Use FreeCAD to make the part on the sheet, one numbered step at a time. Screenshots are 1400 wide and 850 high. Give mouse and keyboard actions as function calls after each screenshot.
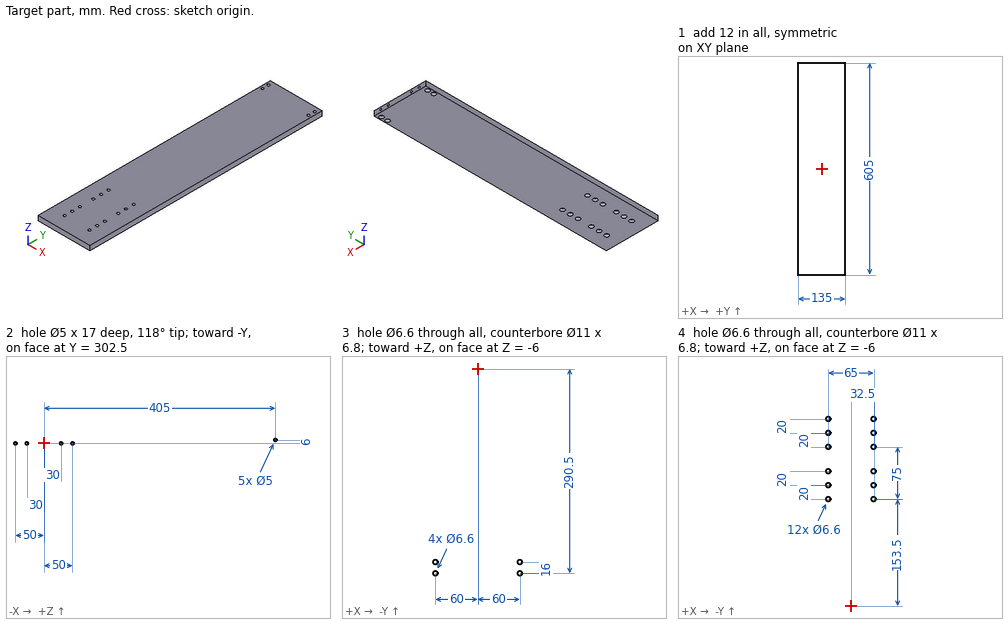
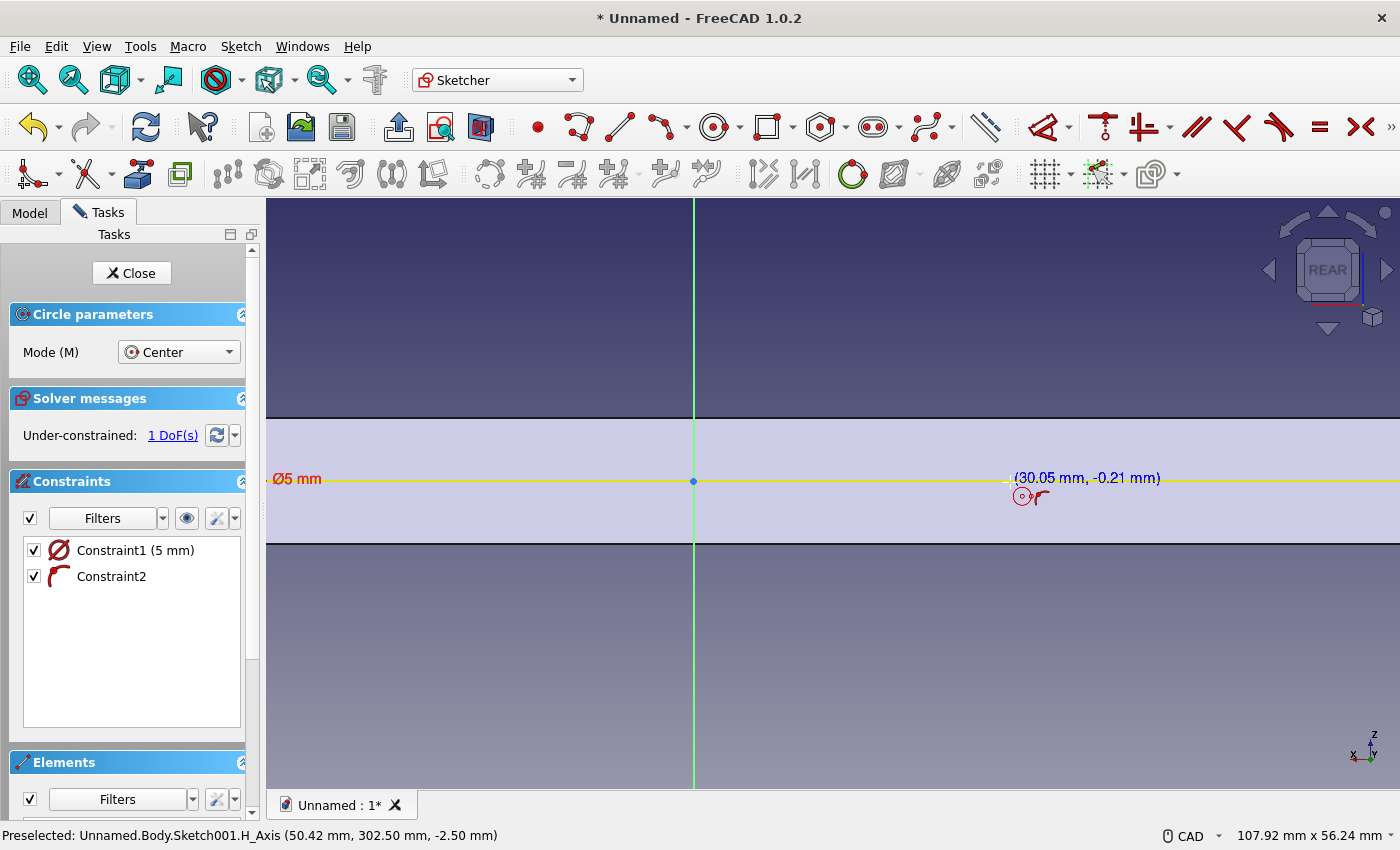
scroll(484, 500, down, 10)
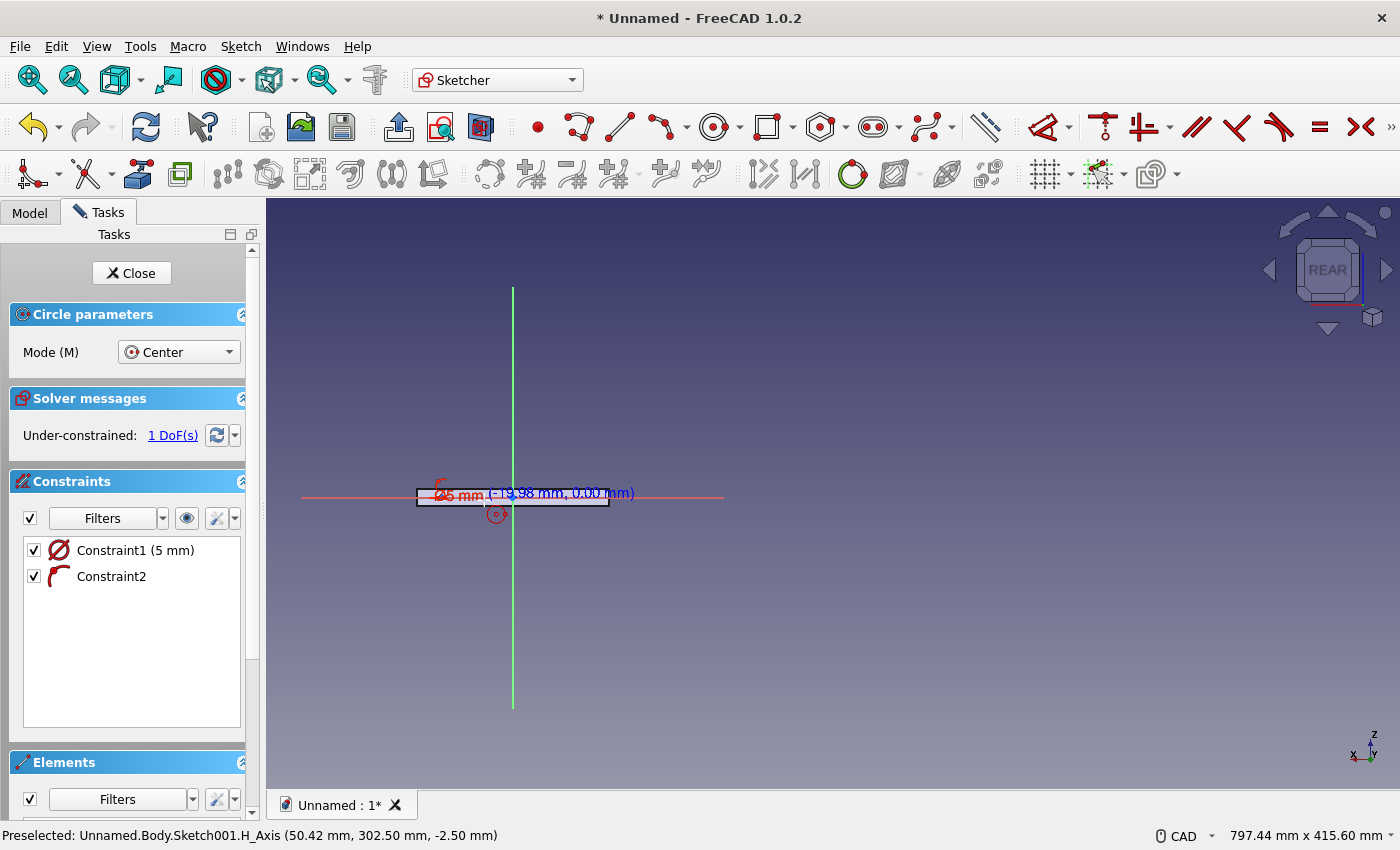
click(555, 498)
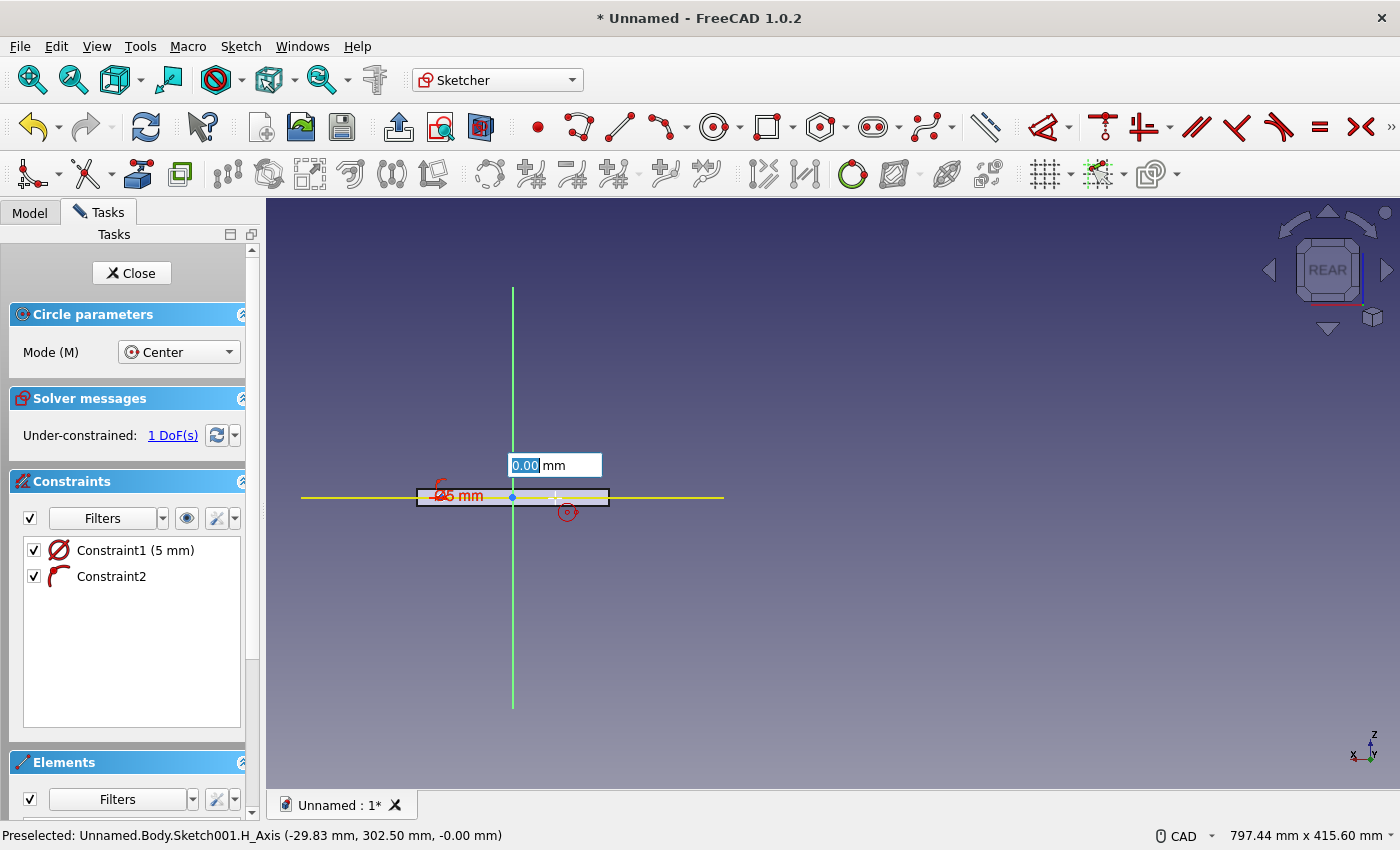
scroll(554, 501, up, 8)
move(553, 500)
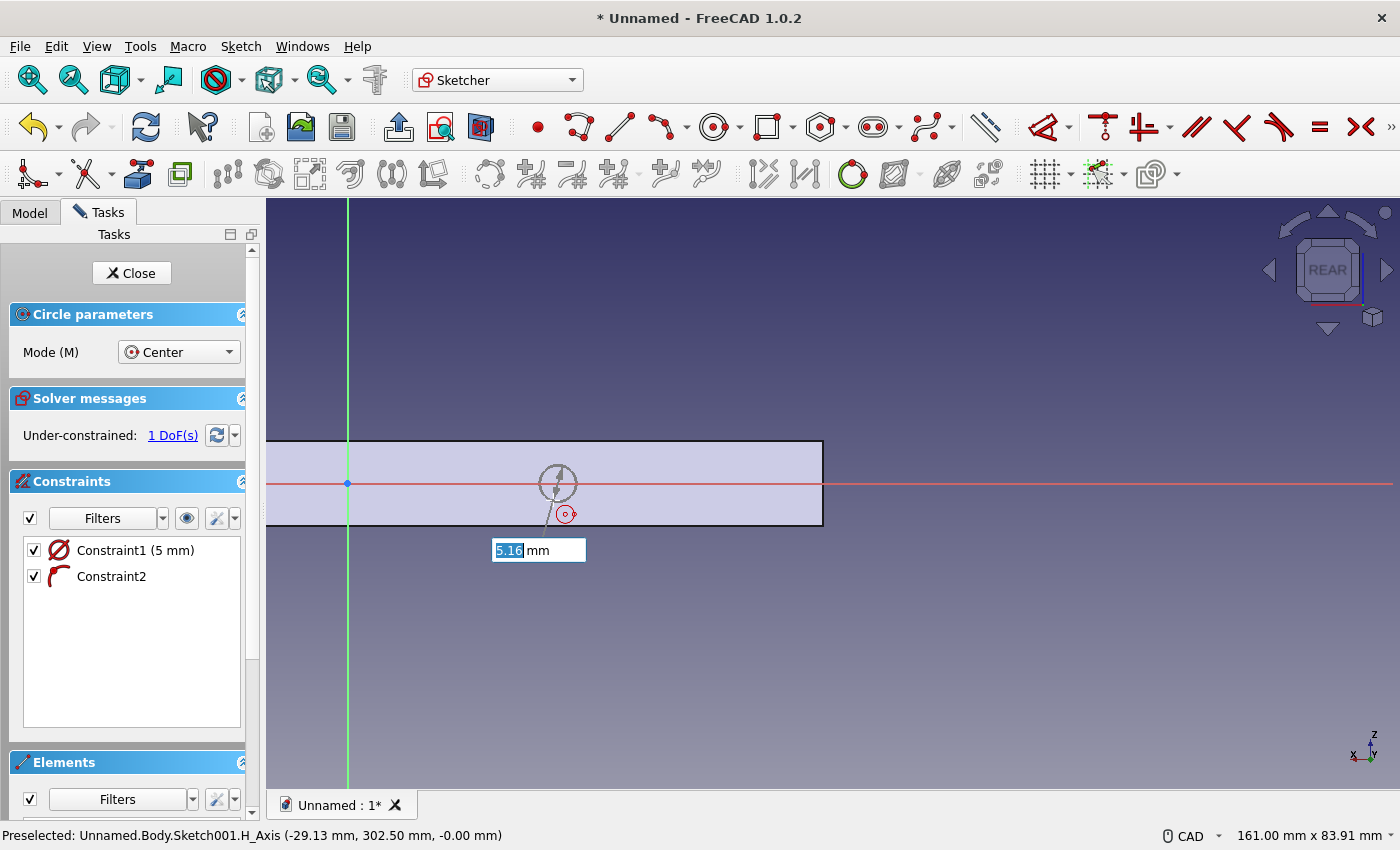
text(5)
key(Return)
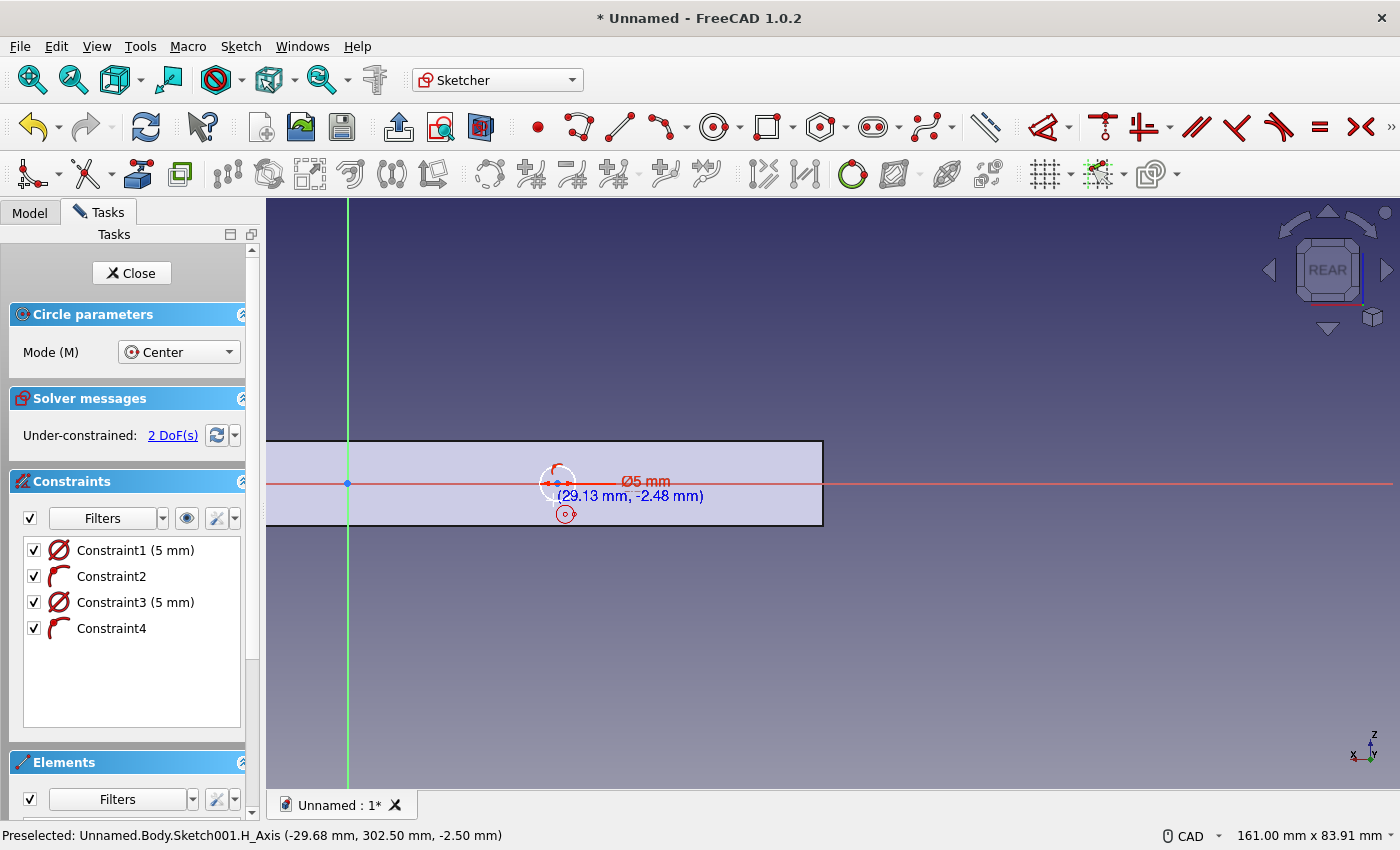
scroll(554, 501, down, 8)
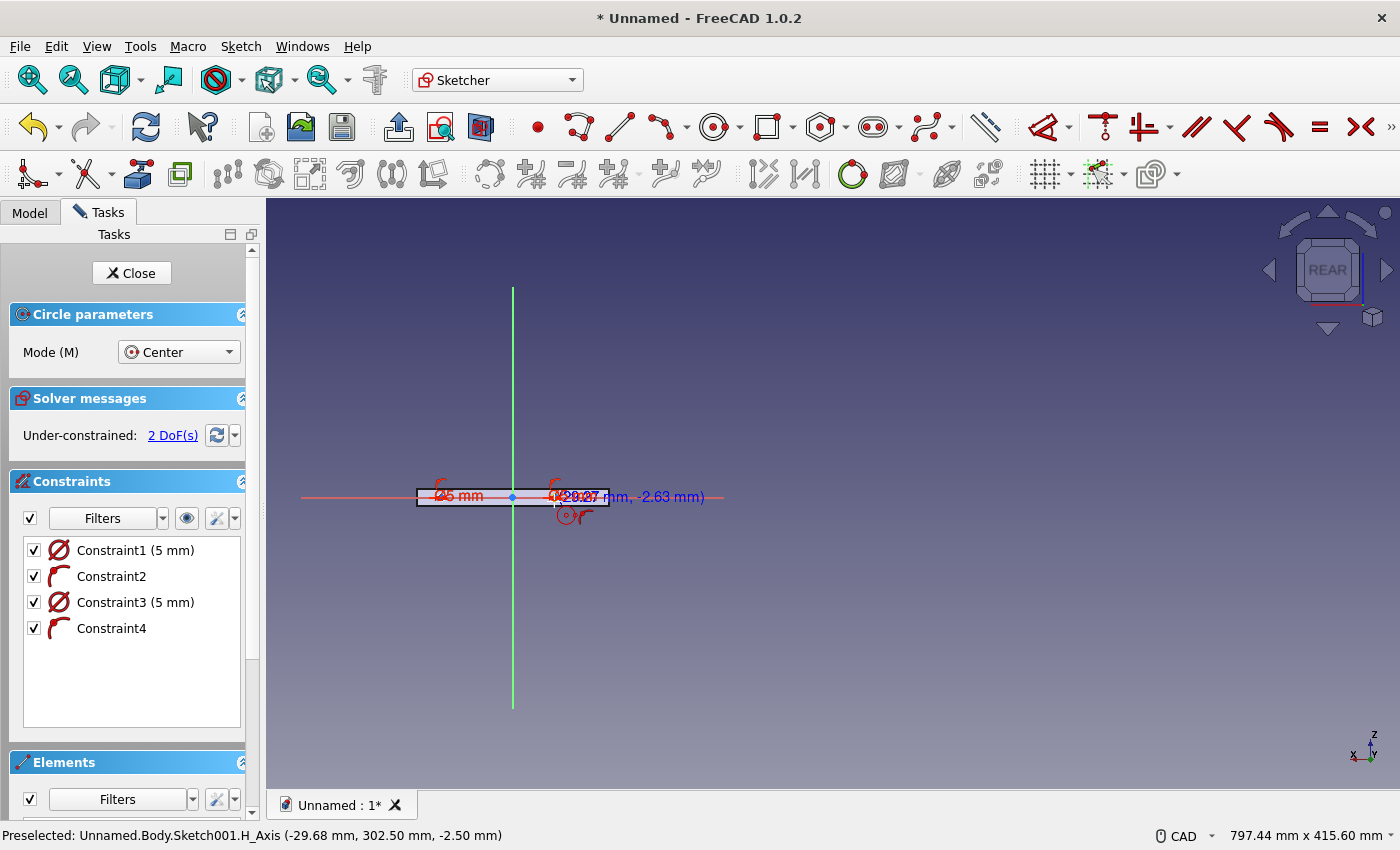
scroll(470, 498, up, 10)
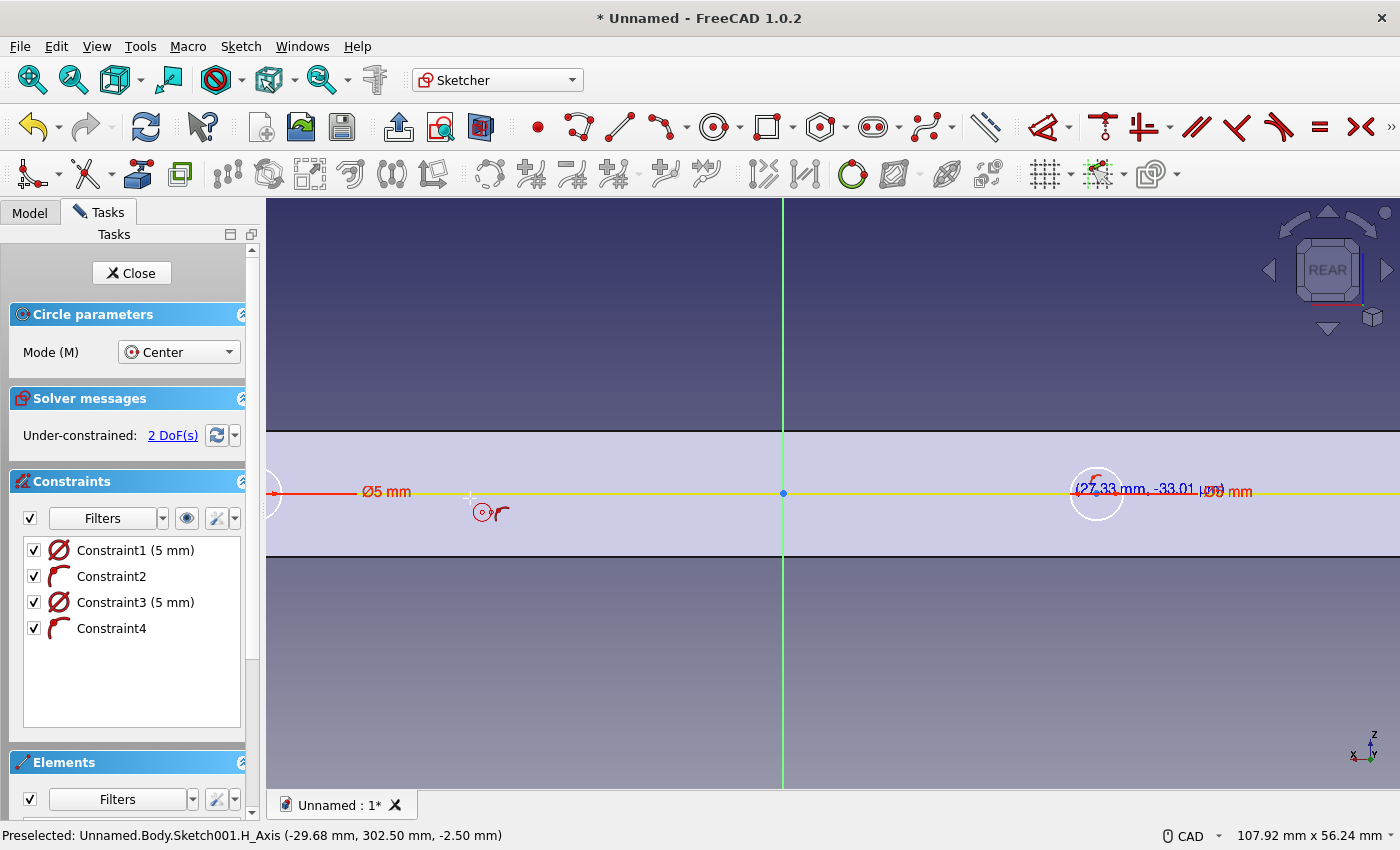
scroll(470, 498, down, 10)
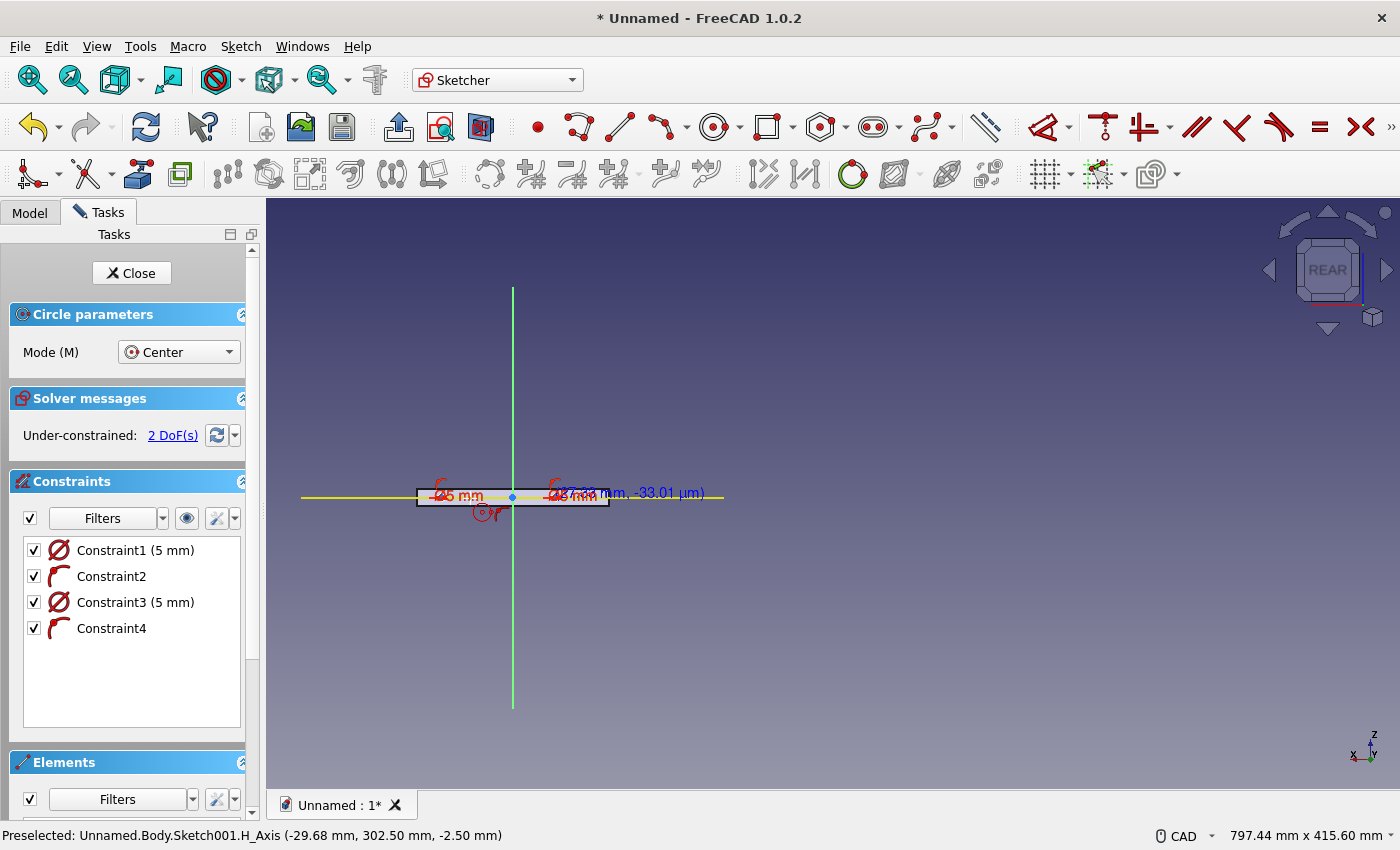
click(470, 498)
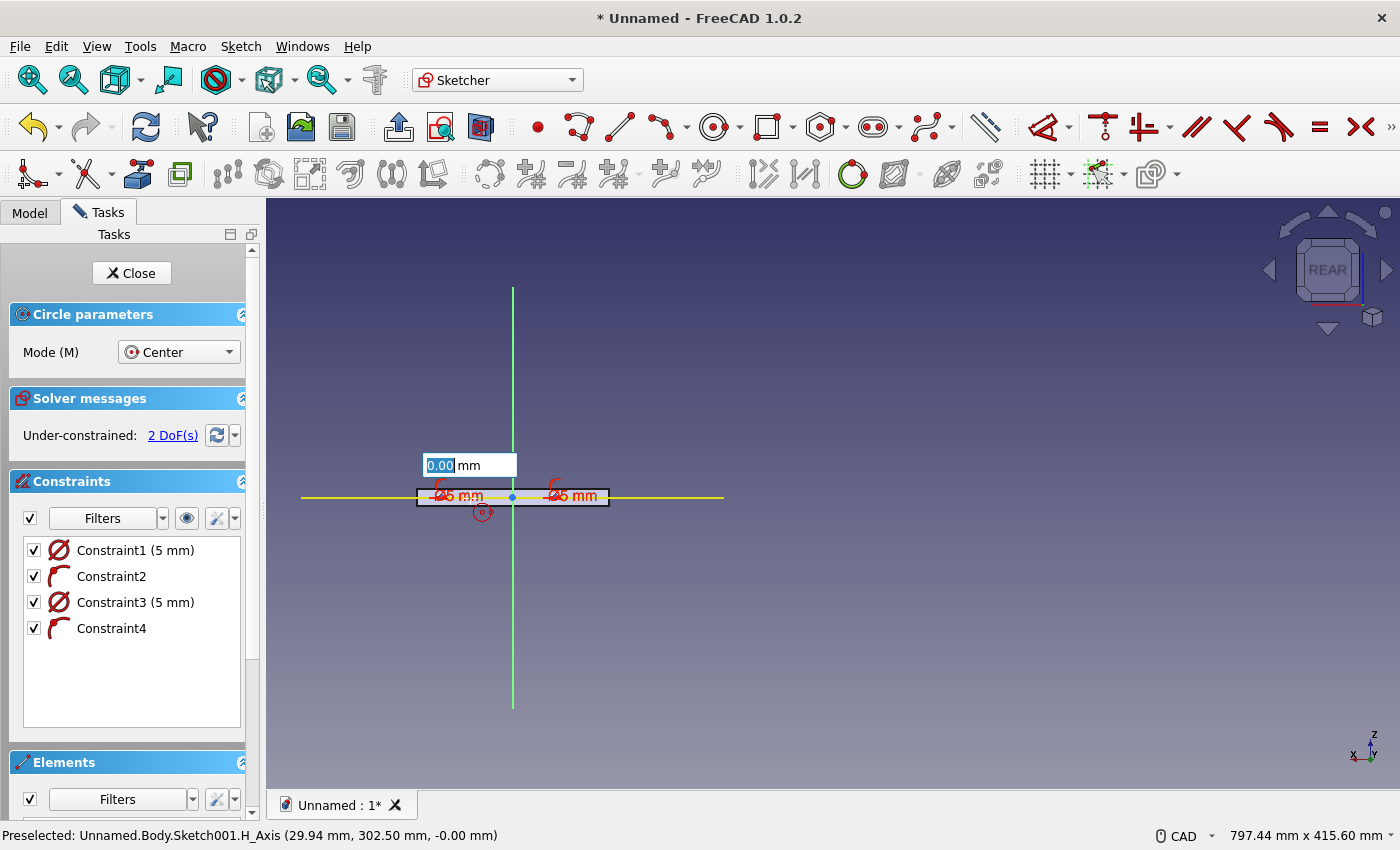
scroll(469, 501, up, 8)
move(467, 500)